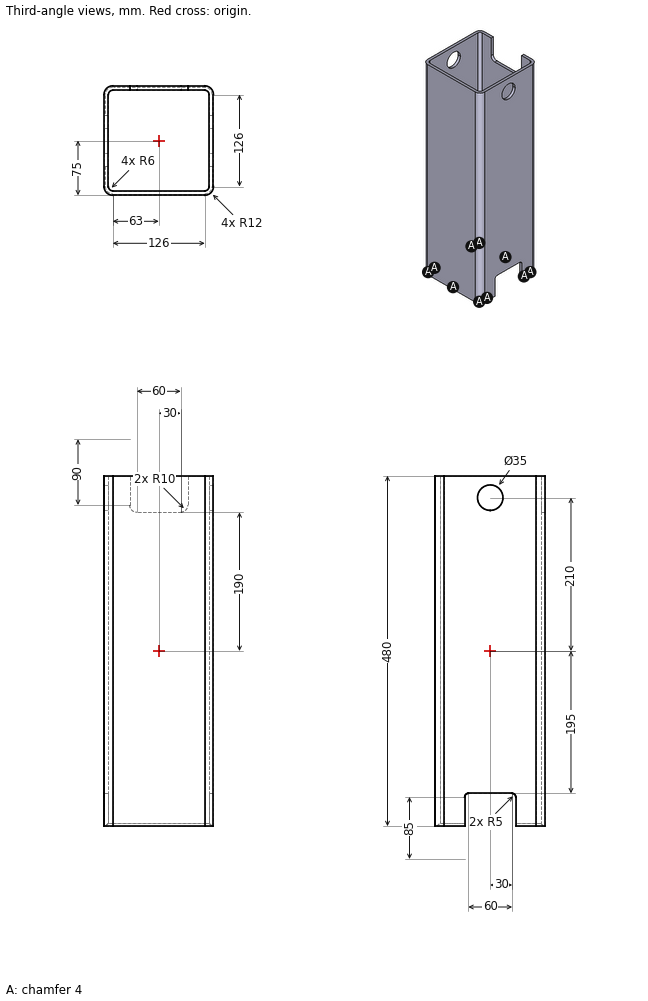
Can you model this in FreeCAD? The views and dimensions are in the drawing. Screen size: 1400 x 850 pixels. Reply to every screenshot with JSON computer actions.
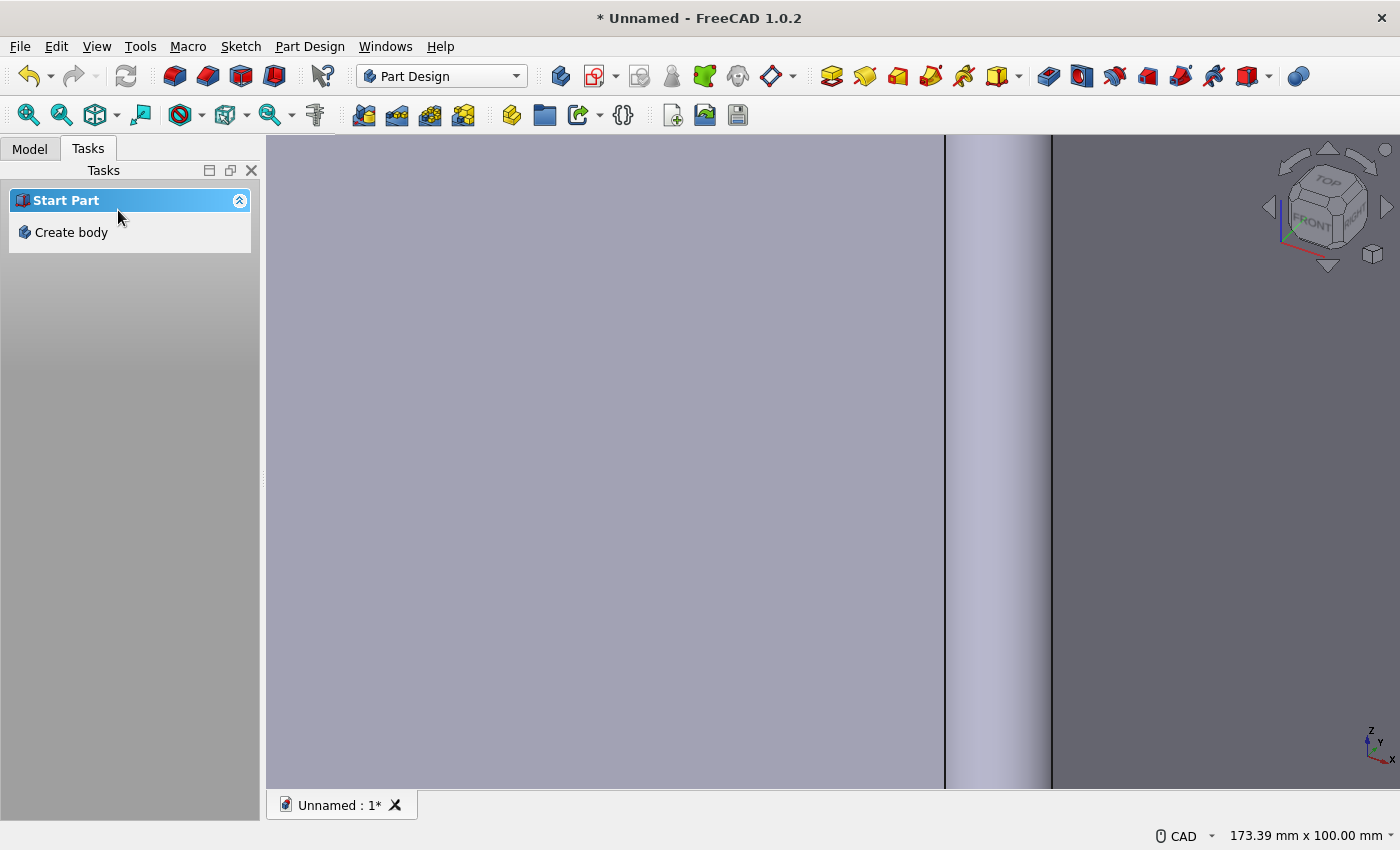
{"action": "left_click", "coordinate": [29, 116]}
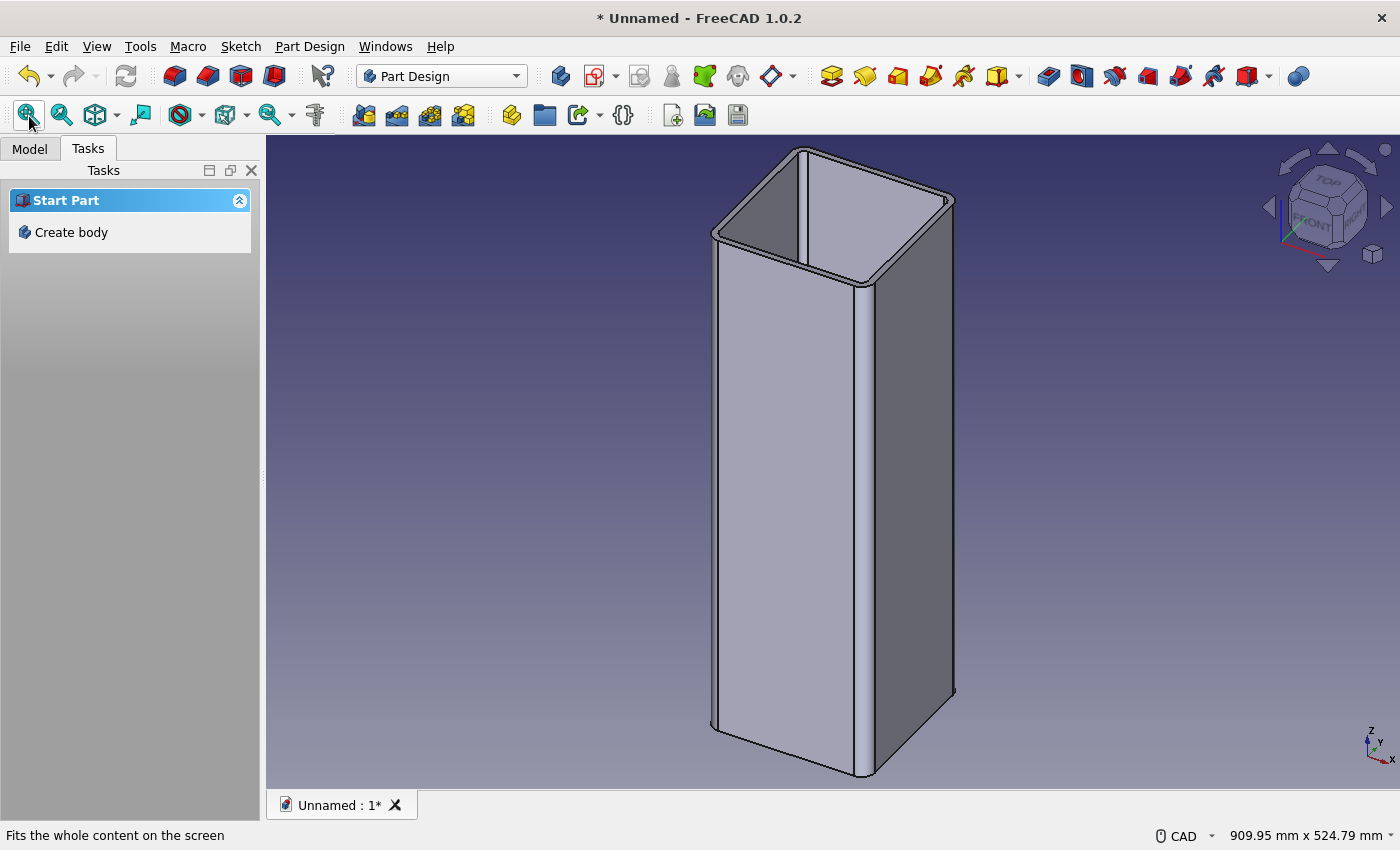
{"action": "left_click", "coordinate": [594, 76]}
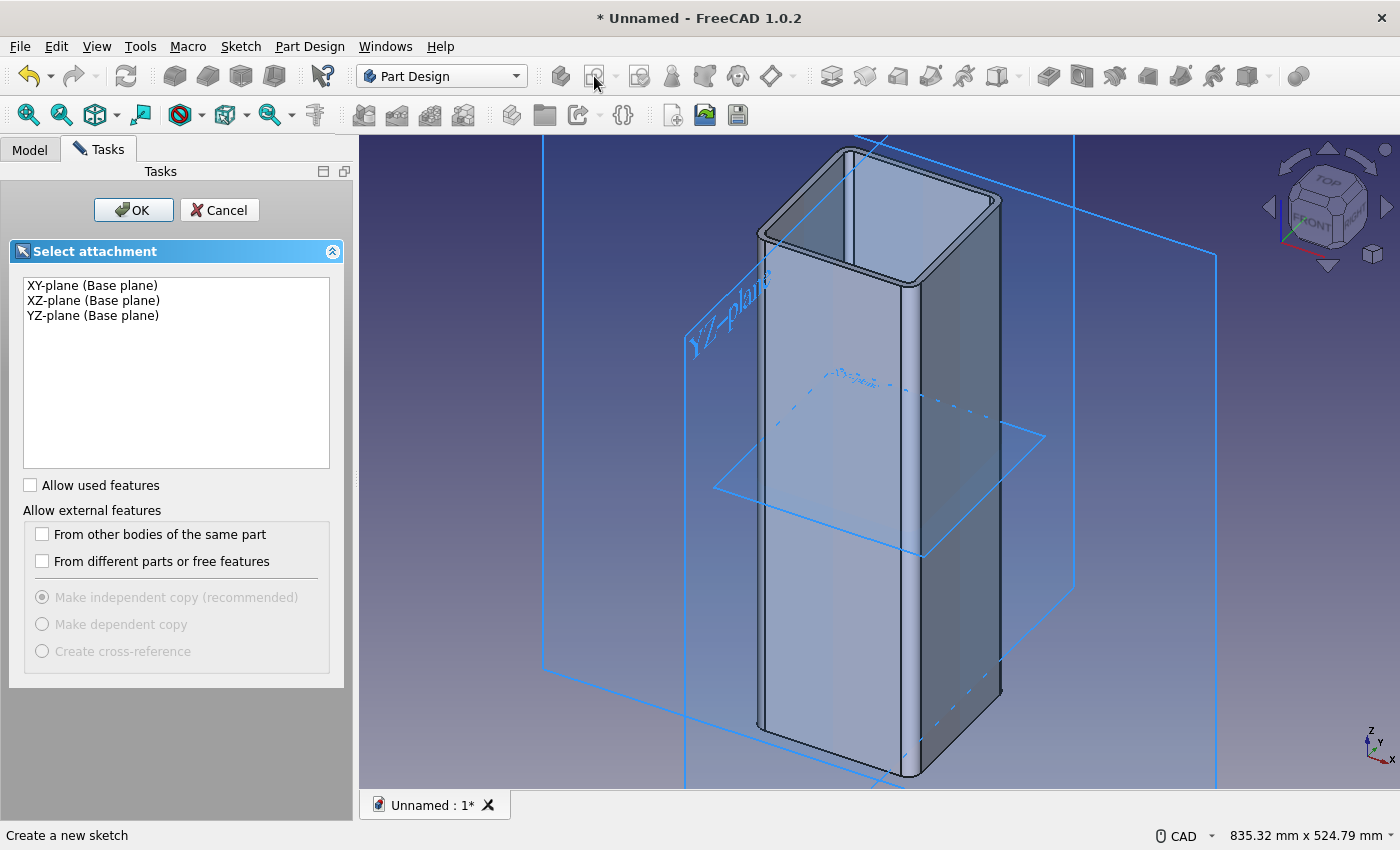
{"action": "left_click", "coordinate": [84, 300]}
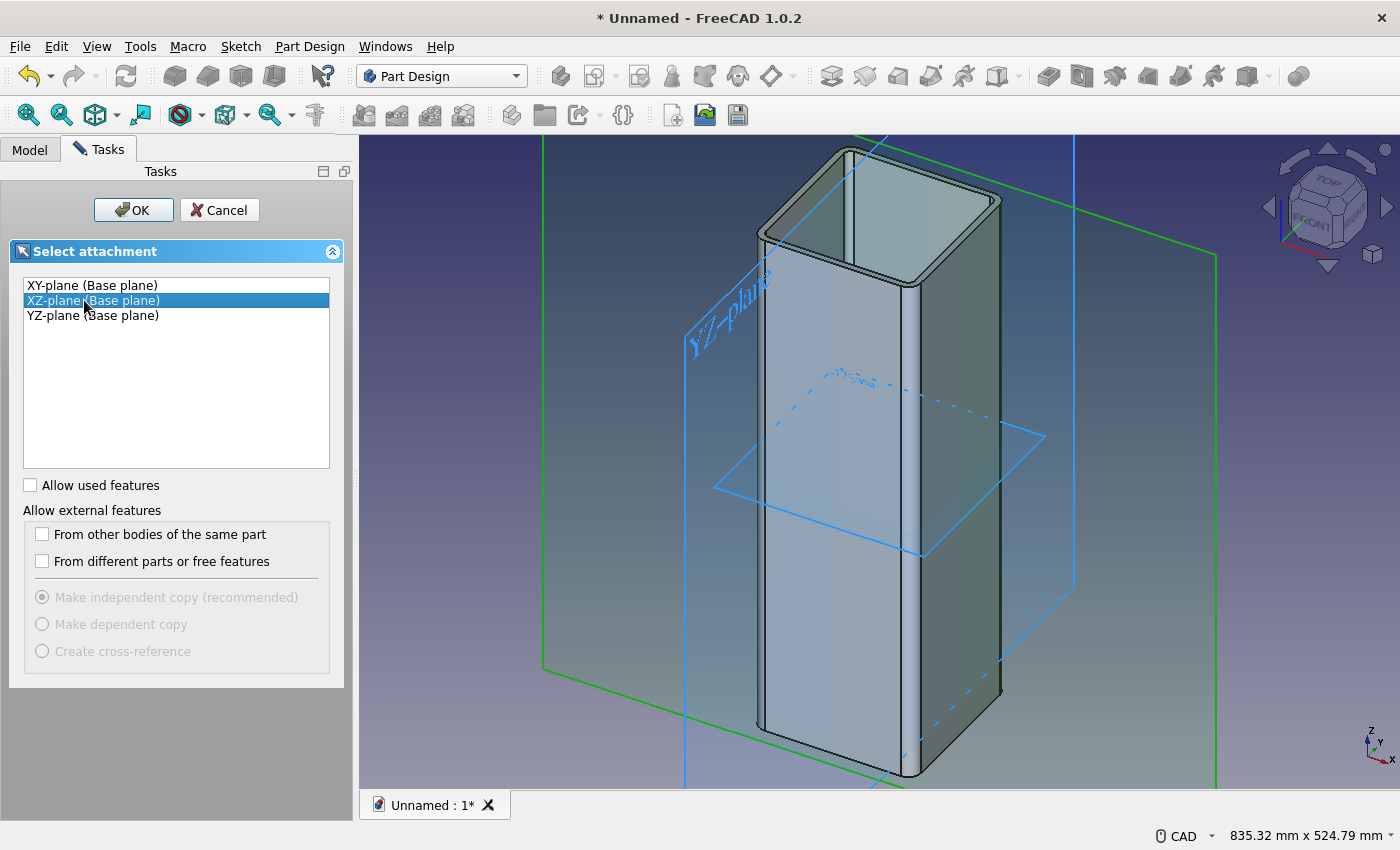
{"action": "left_click", "coordinate": [134, 210]}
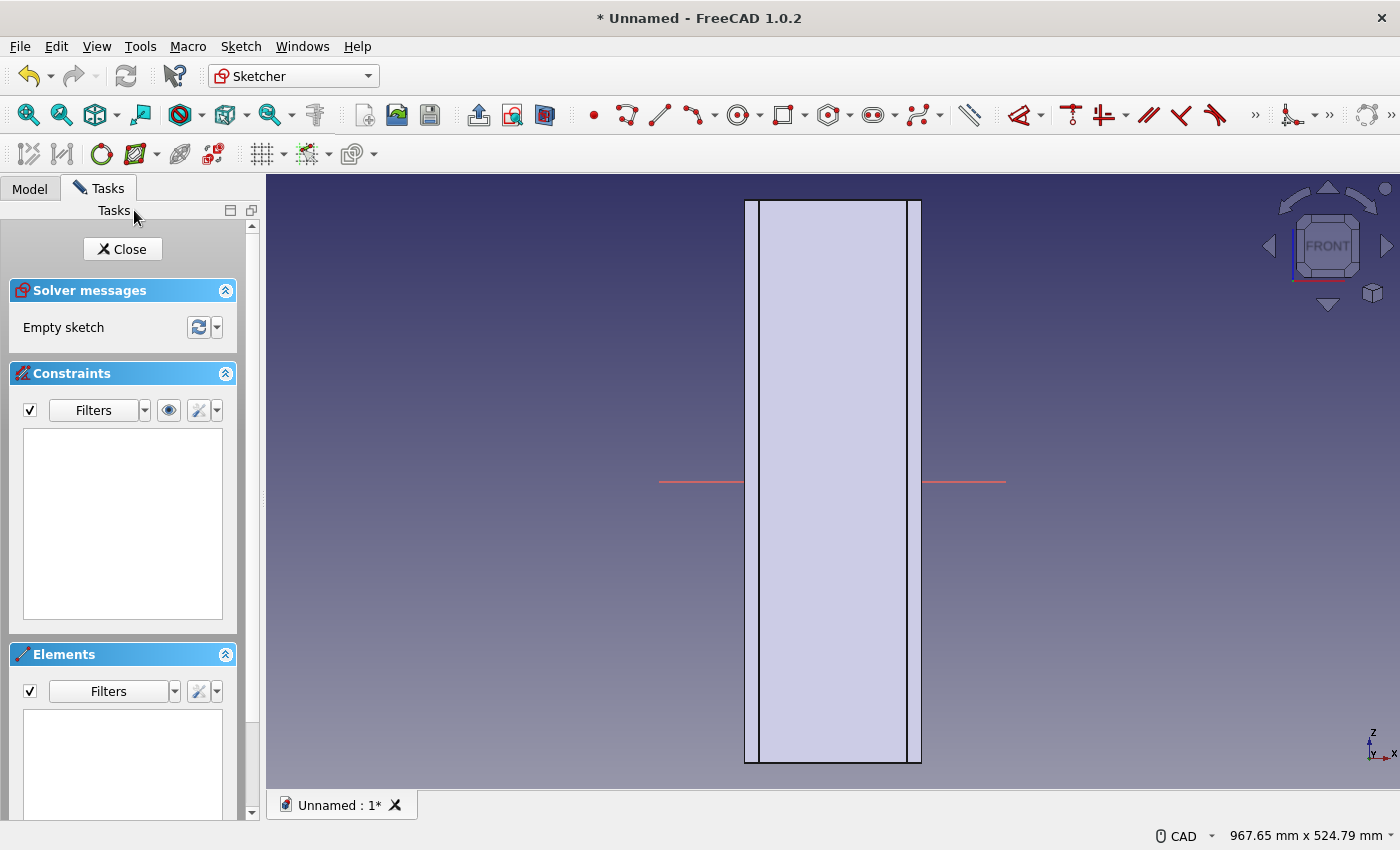
{"action": "key", "text": "q s"}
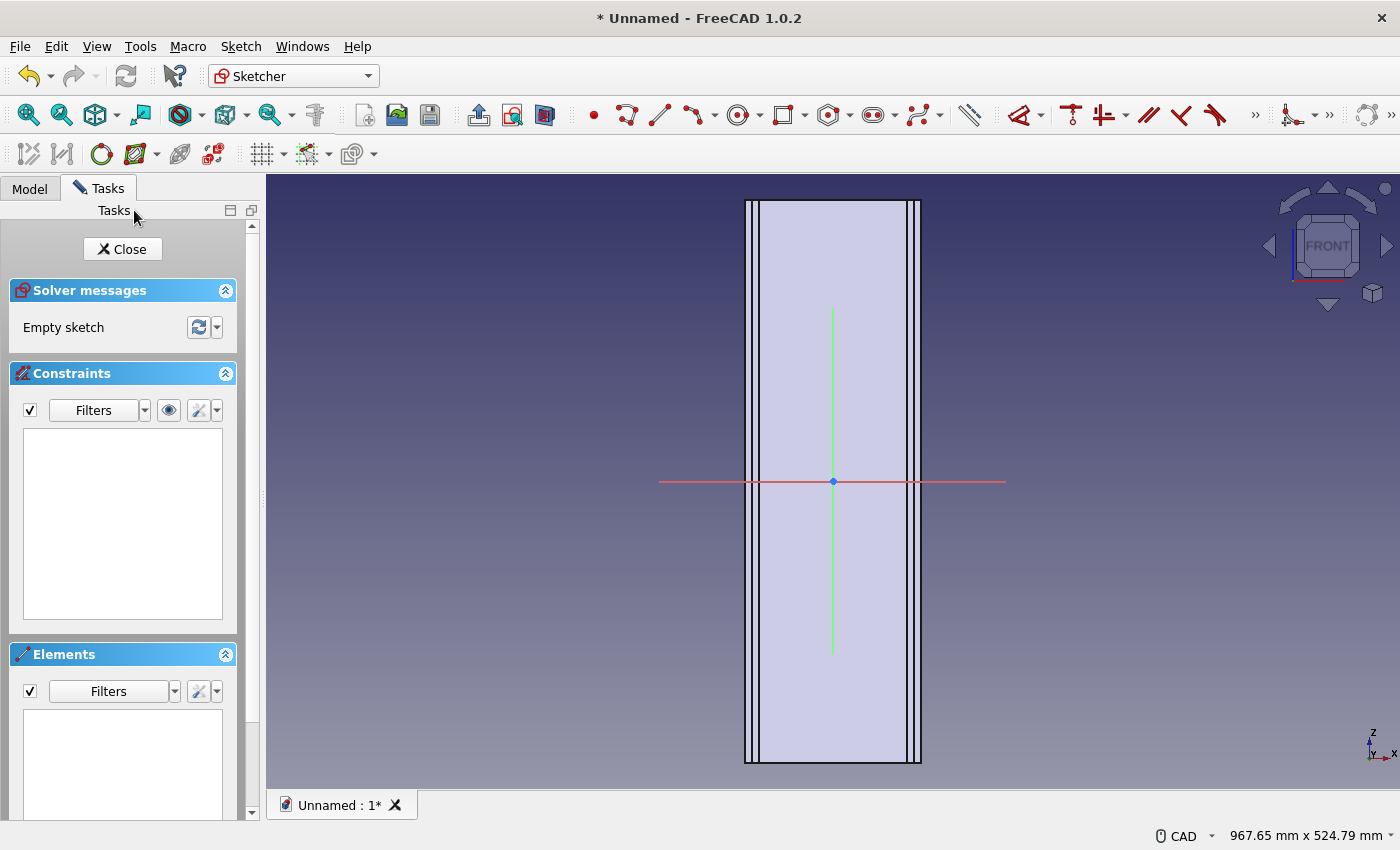
{"action": "scroll", "coordinate": [764, 482], "scroll_direction": "down", "scroll_amount": 5}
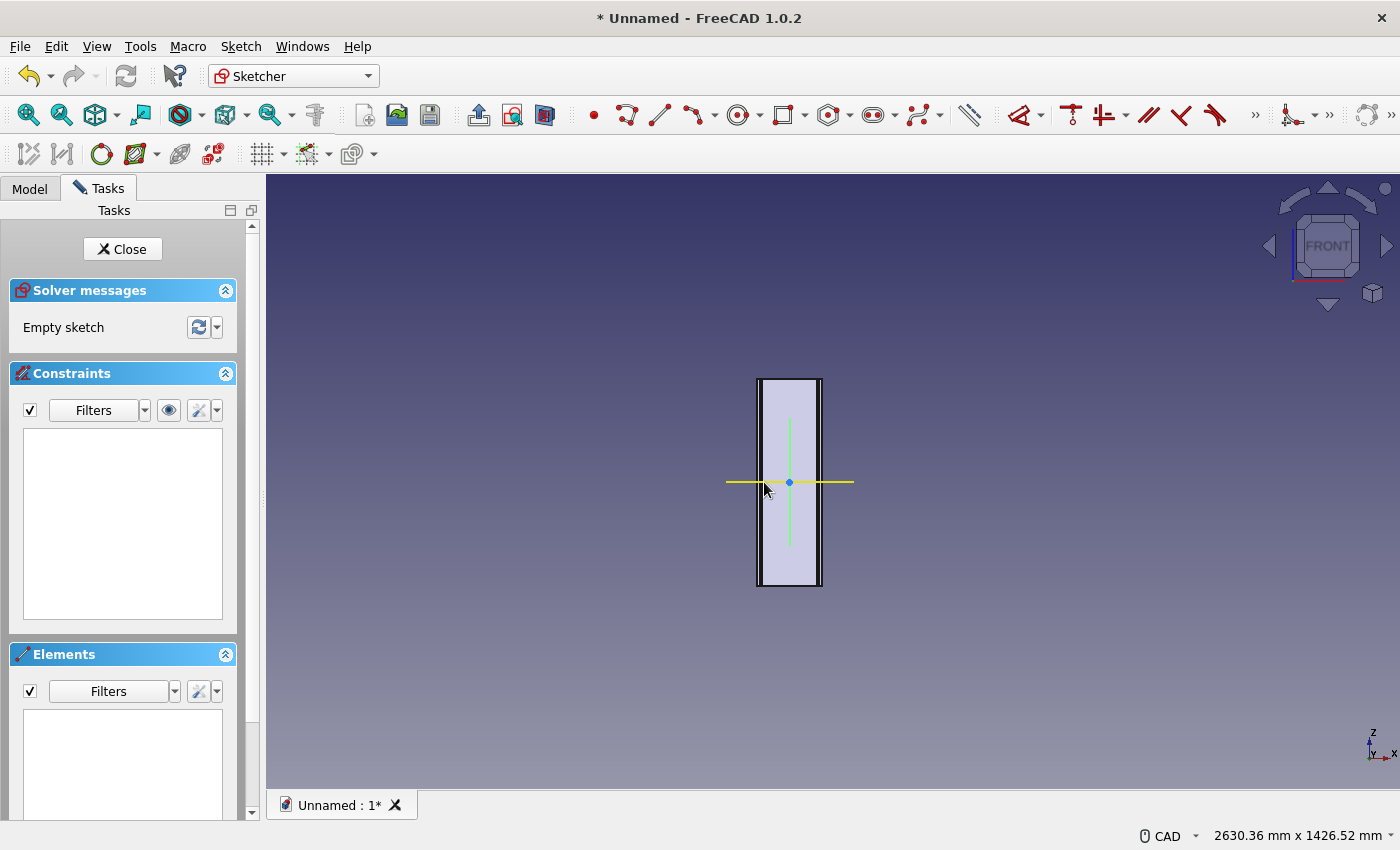
{"action": "scroll", "coordinate": [793, 366], "scroll_direction": "up", "scroll_amount": 11}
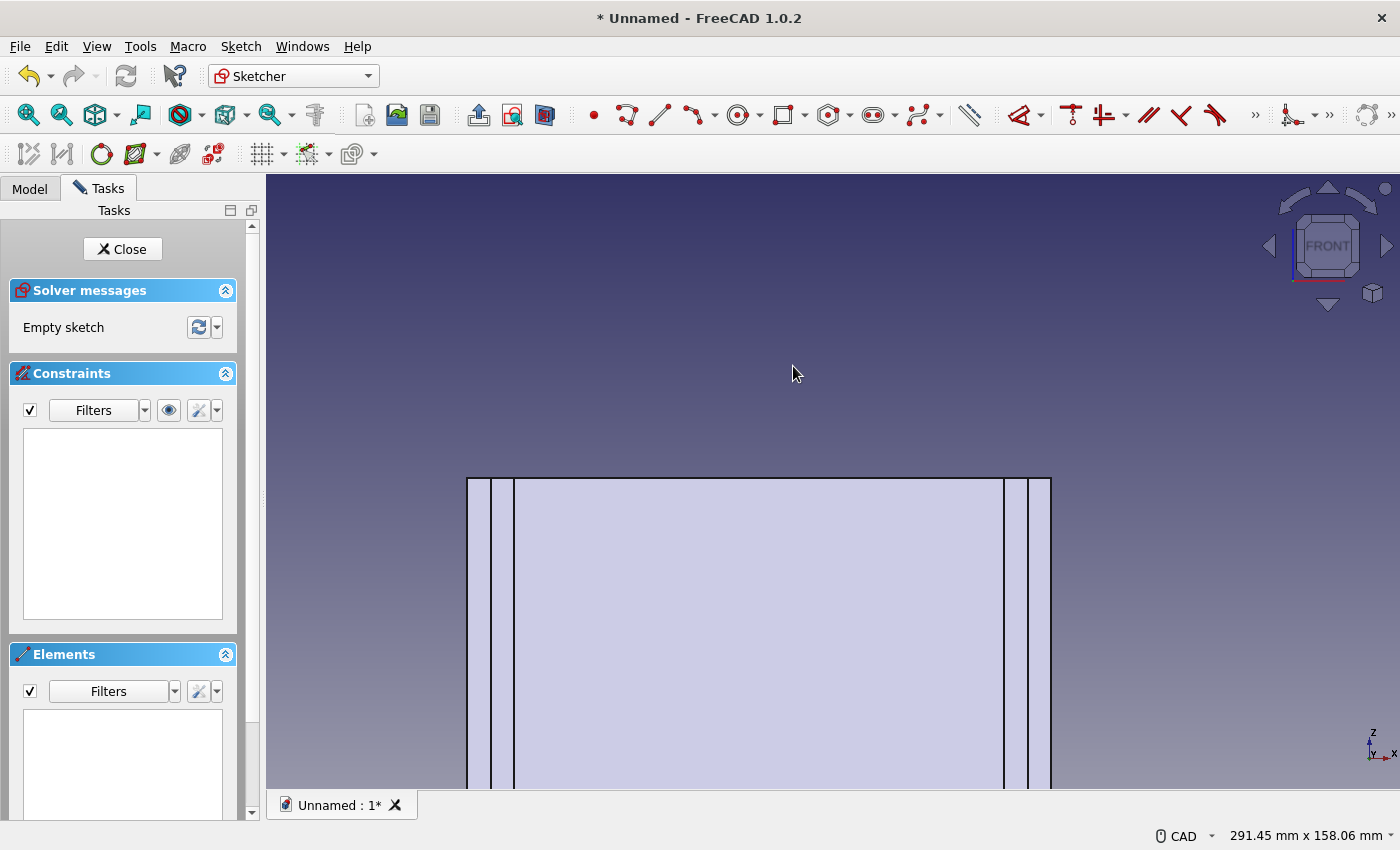
{"action": "left_click", "coordinate": [660, 116]}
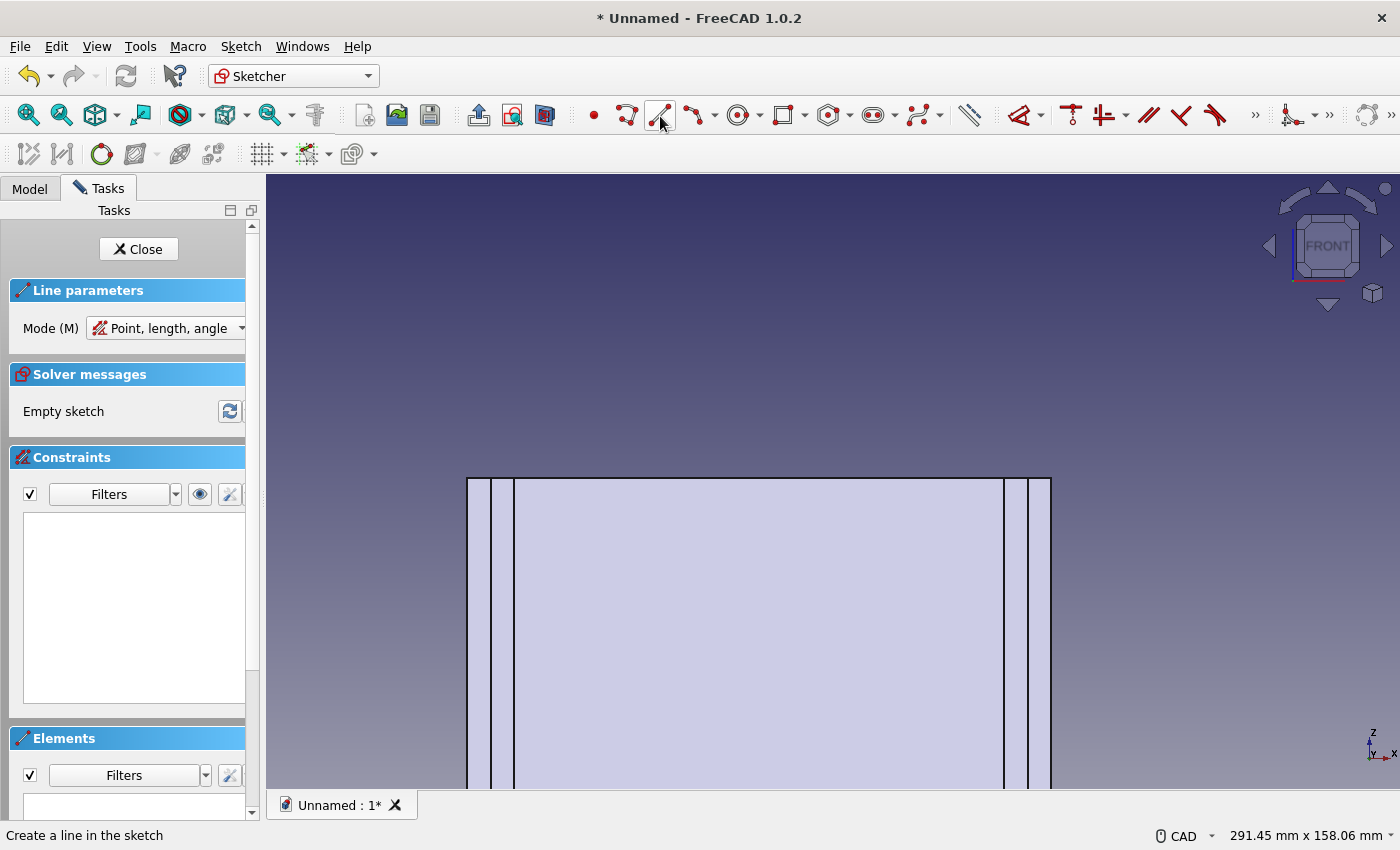
{"action": "left_click", "coordinate": [876, 672]}
{"action": "left_click", "coordinate": [642, 672]}